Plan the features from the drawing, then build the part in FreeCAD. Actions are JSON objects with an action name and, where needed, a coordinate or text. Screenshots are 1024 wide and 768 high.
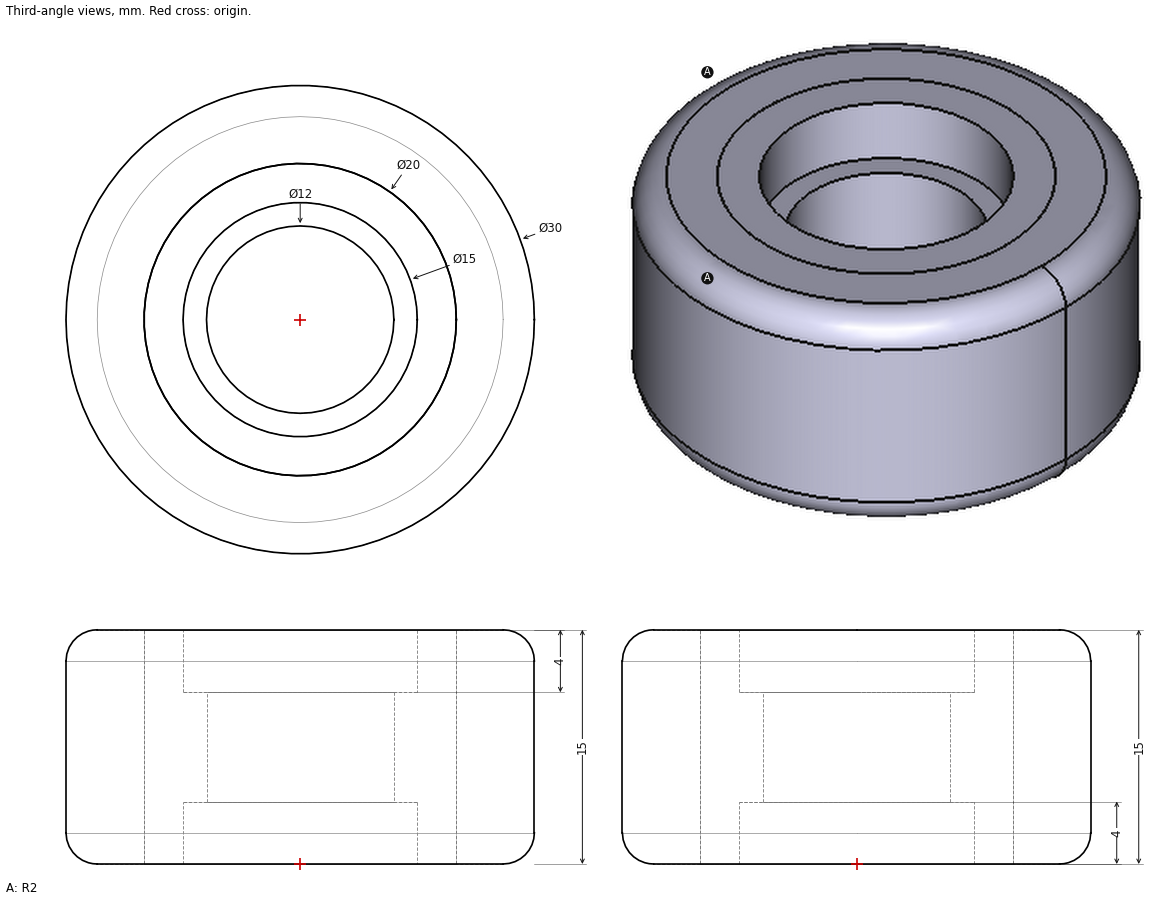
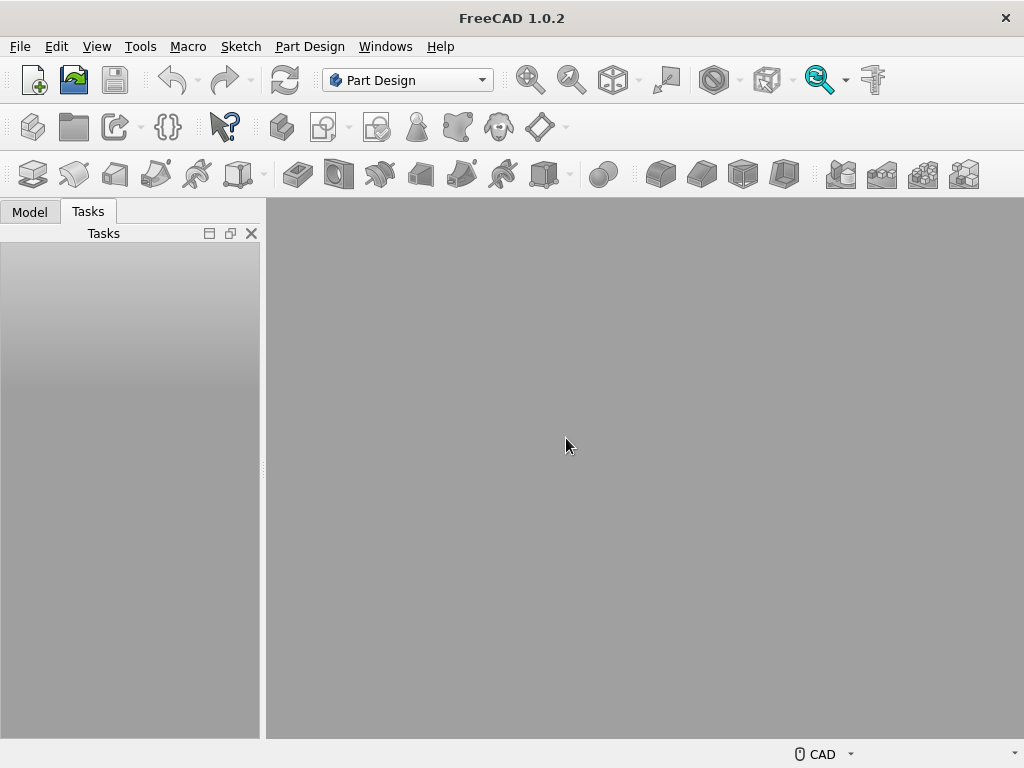
{"action": "key", "text": "ctrl+n"}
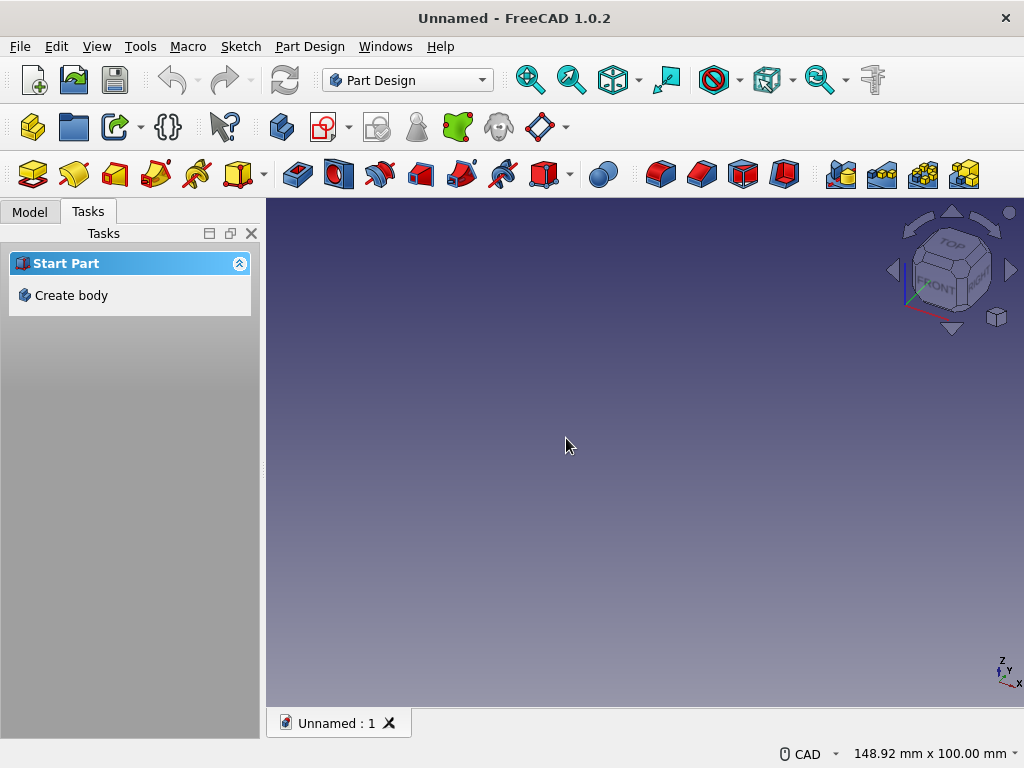
{"action": "left_click", "coordinate": [322, 128]}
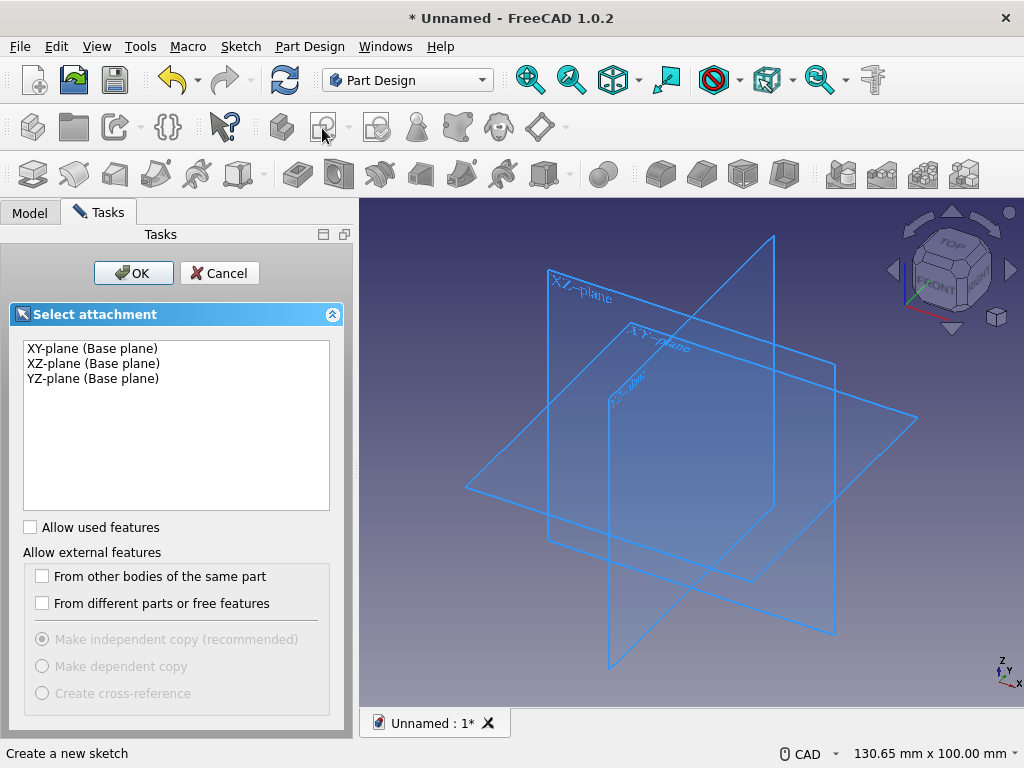
{"action": "left_click", "coordinate": [84, 348]}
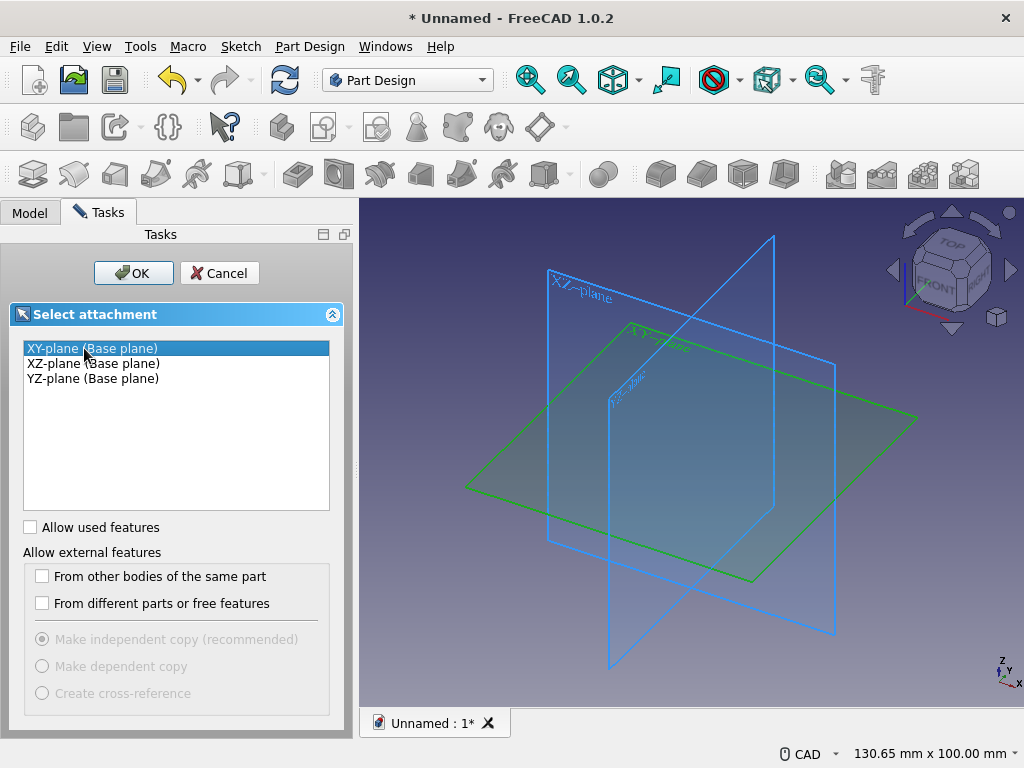
{"action": "left_click", "coordinate": [134, 273]}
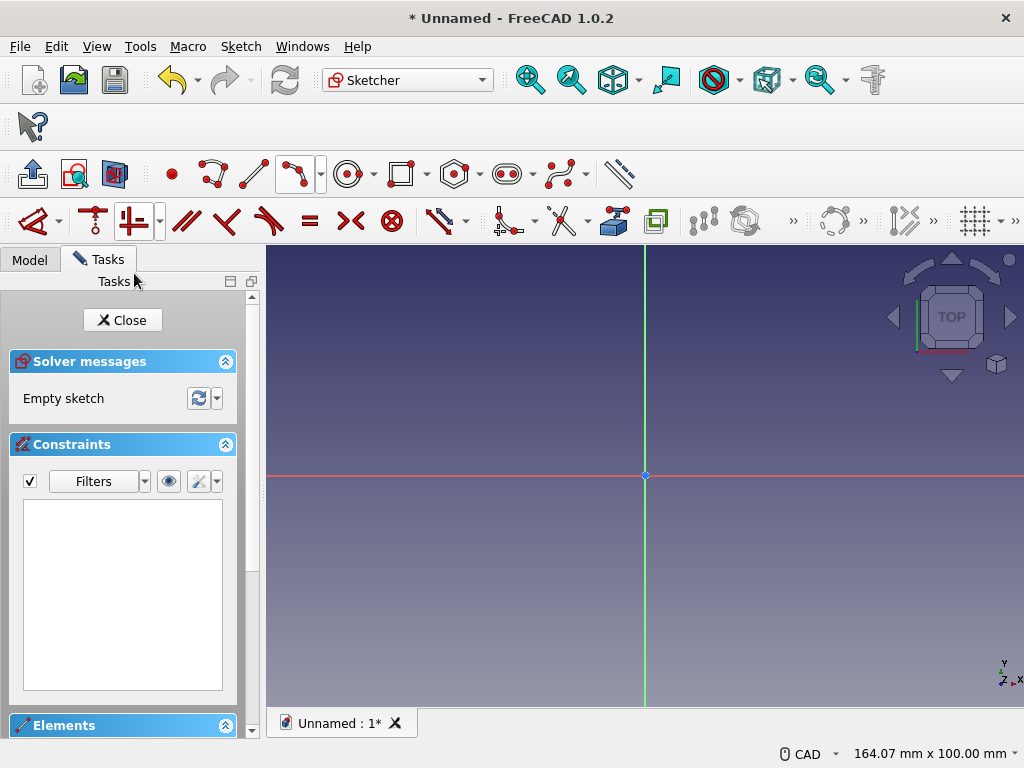
{"action": "scroll", "coordinate": [675, 476], "scroll_direction": "up", "scroll_amount": 6}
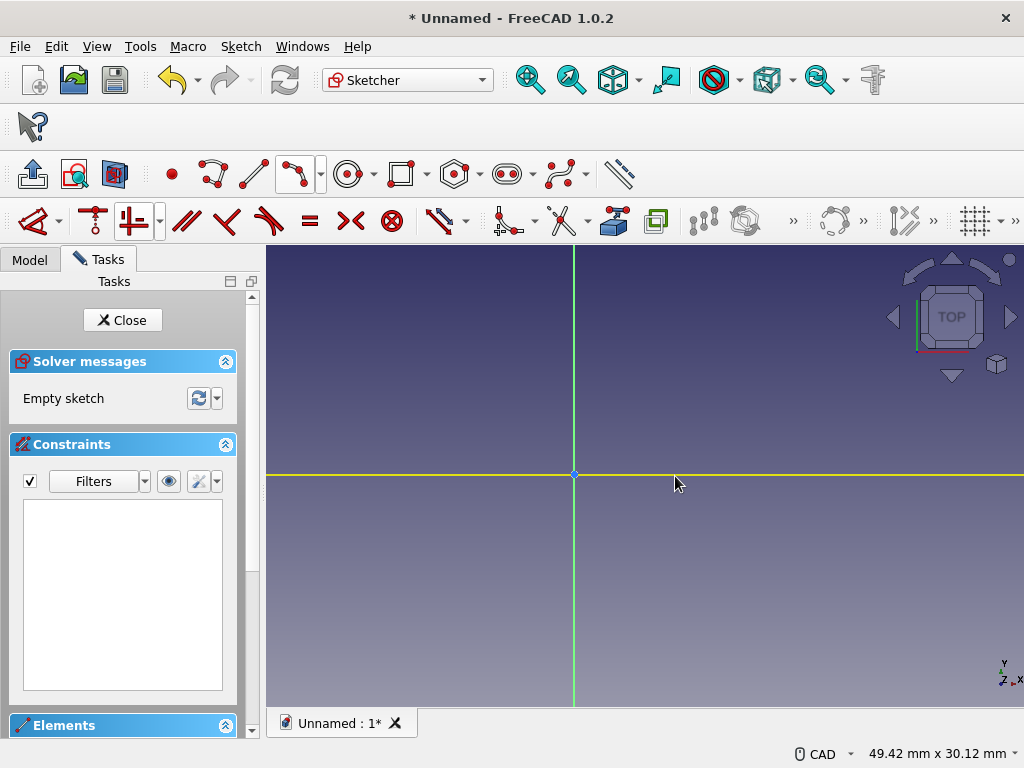
{"action": "key", "text": "g c"}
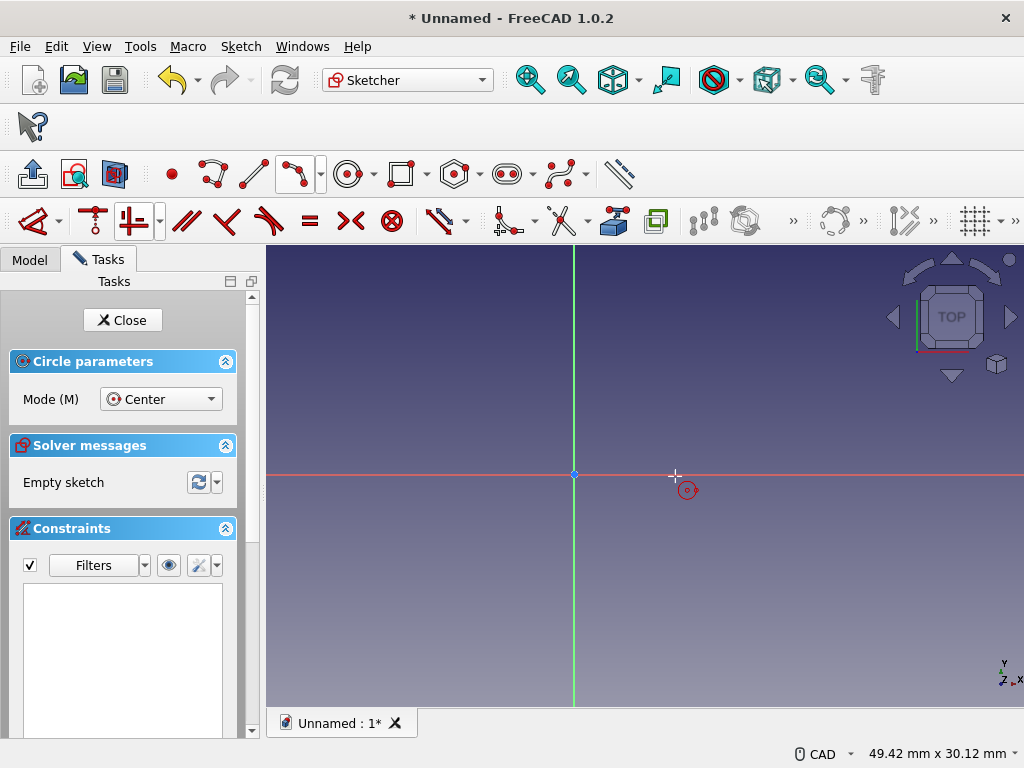
{"action": "left_click", "coordinate": [574, 475]}
{"action": "mouse_move", "coordinate": [683, 366]}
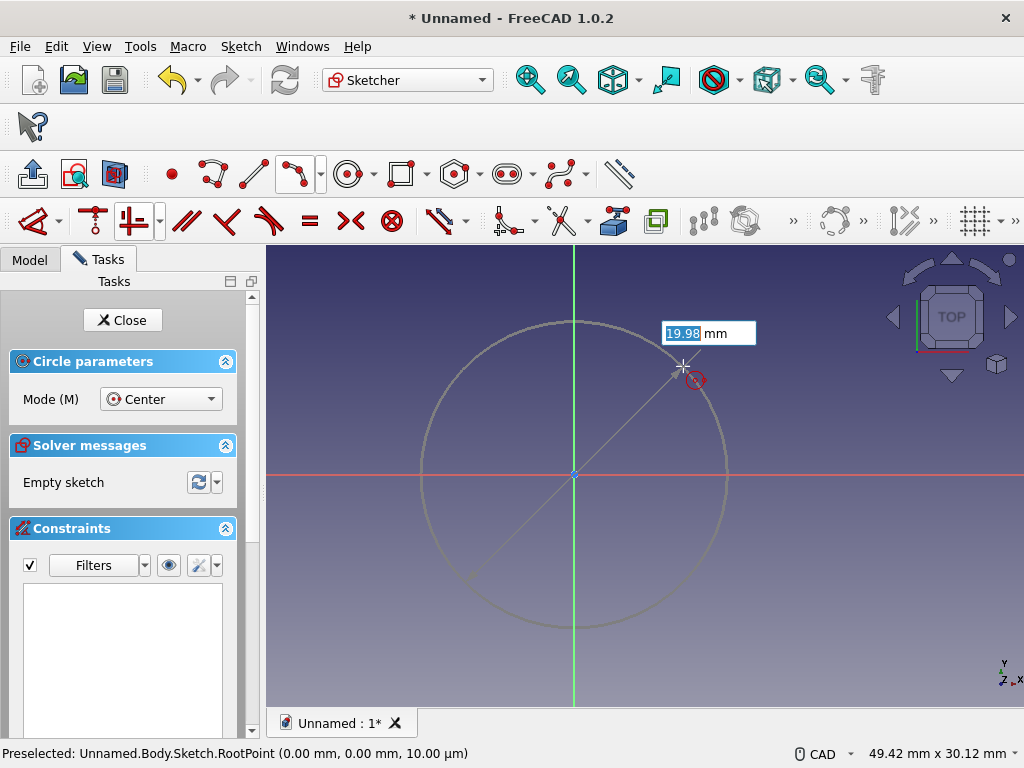
{"action": "type", "text": "20"}
{"action": "key", "text": "Return"}
{"action": "key", "text": "Escape"}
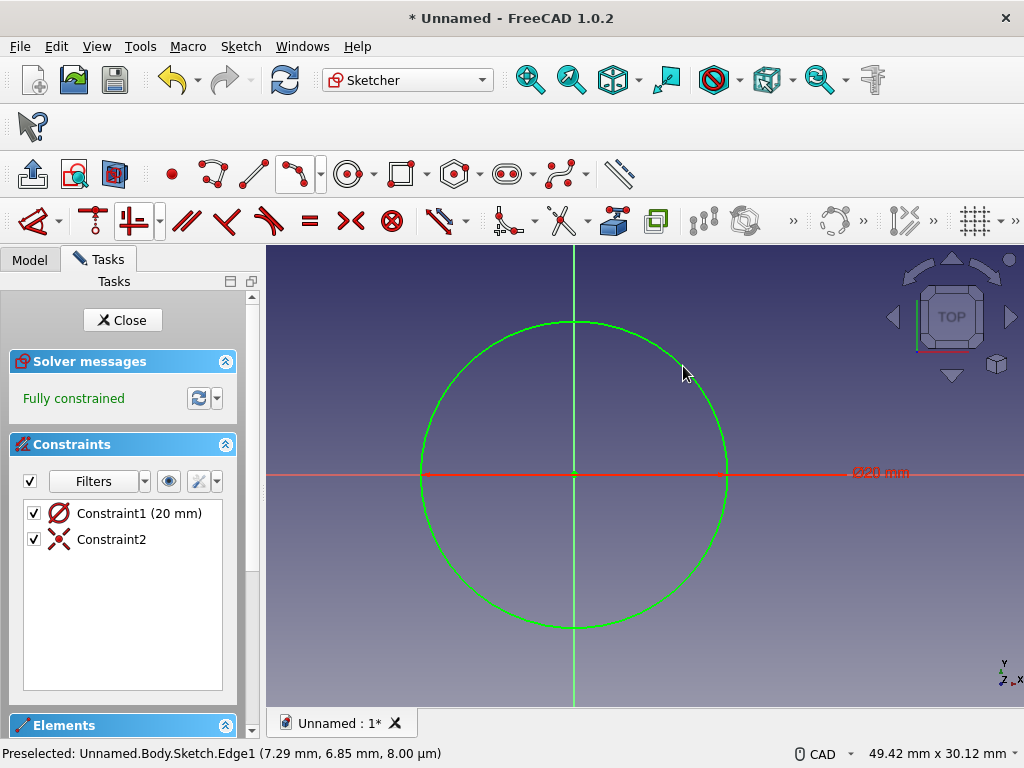
{"action": "left_click", "coordinate": [123, 320]}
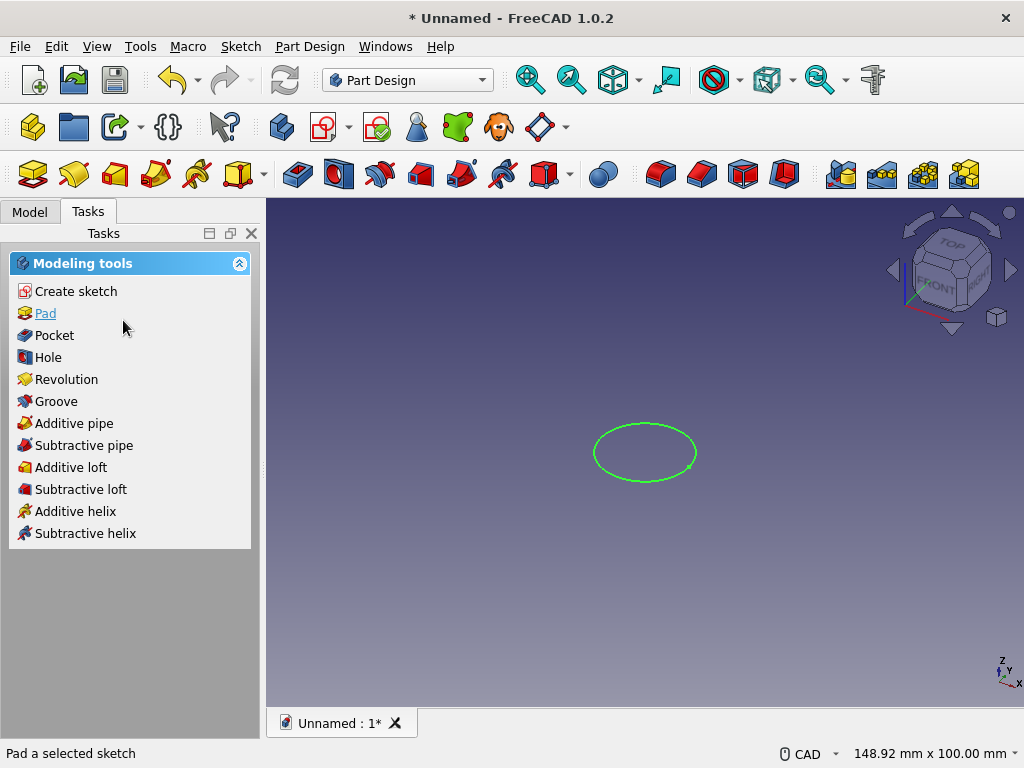
{"action": "left_click", "coordinate": [33, 174]}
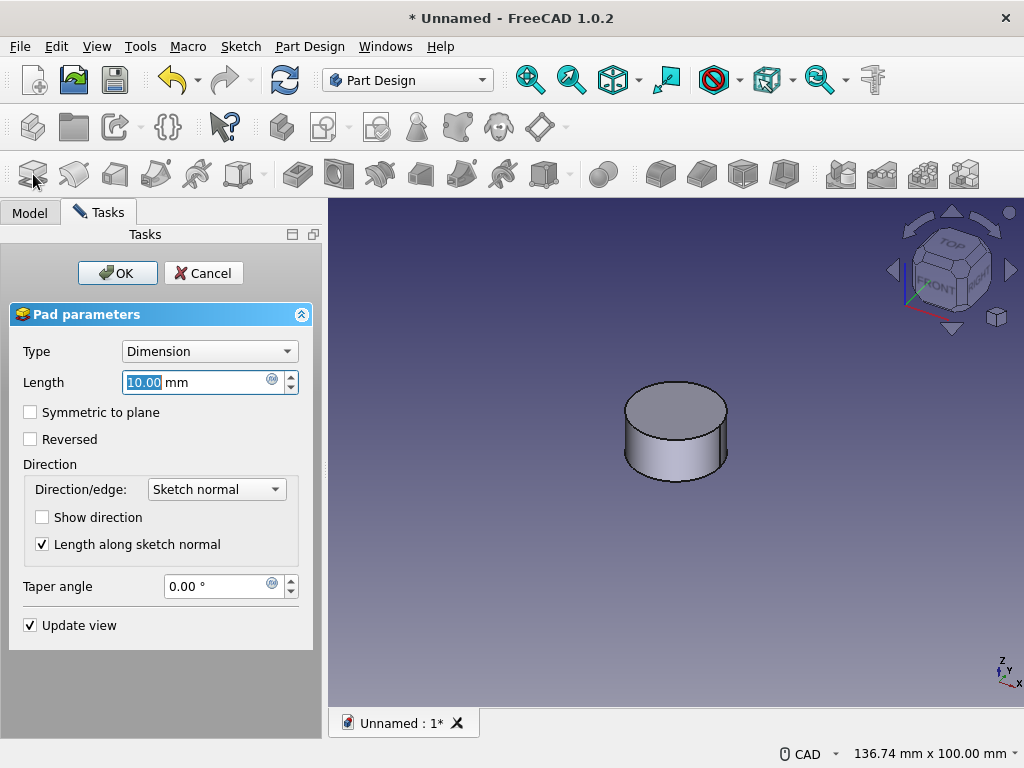
{"action": "type", "text": "15"}
{"action": "key", "text": "Tab"}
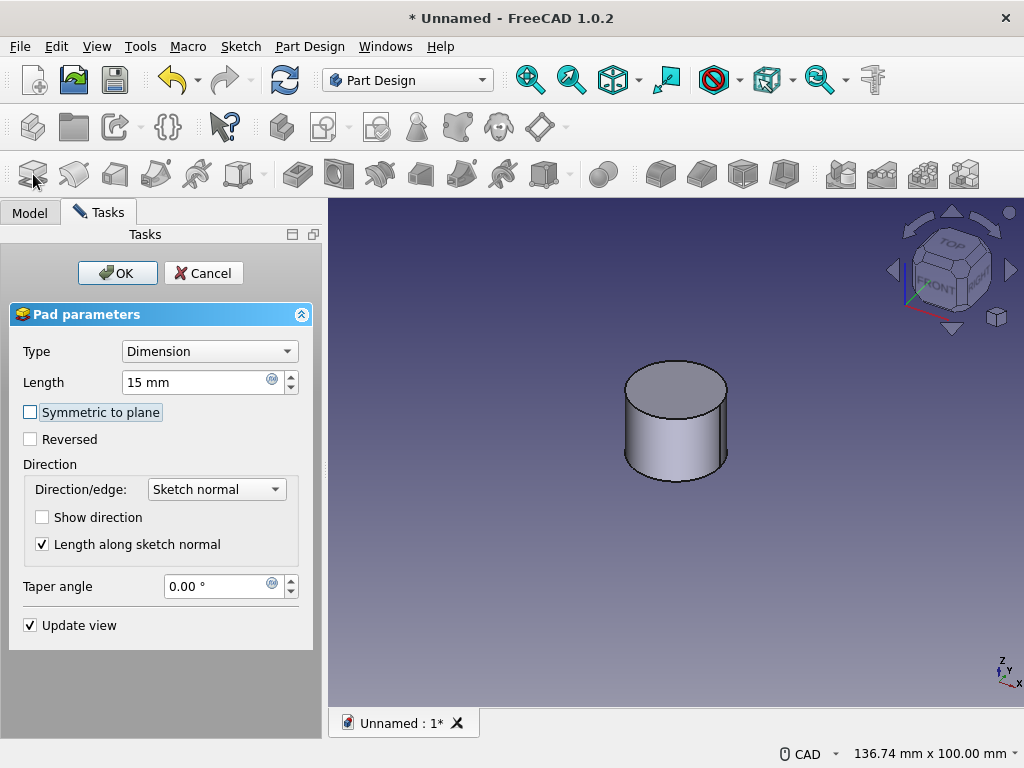
{"action": "left_click", "coordinate": [118, 273]}